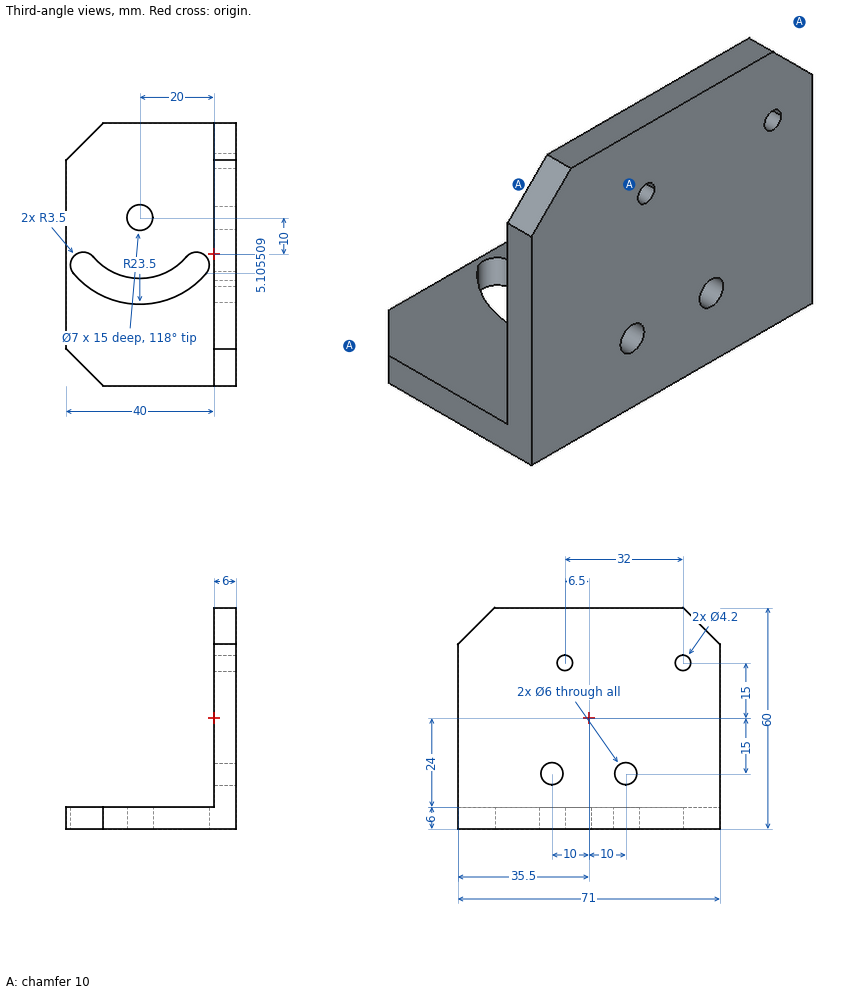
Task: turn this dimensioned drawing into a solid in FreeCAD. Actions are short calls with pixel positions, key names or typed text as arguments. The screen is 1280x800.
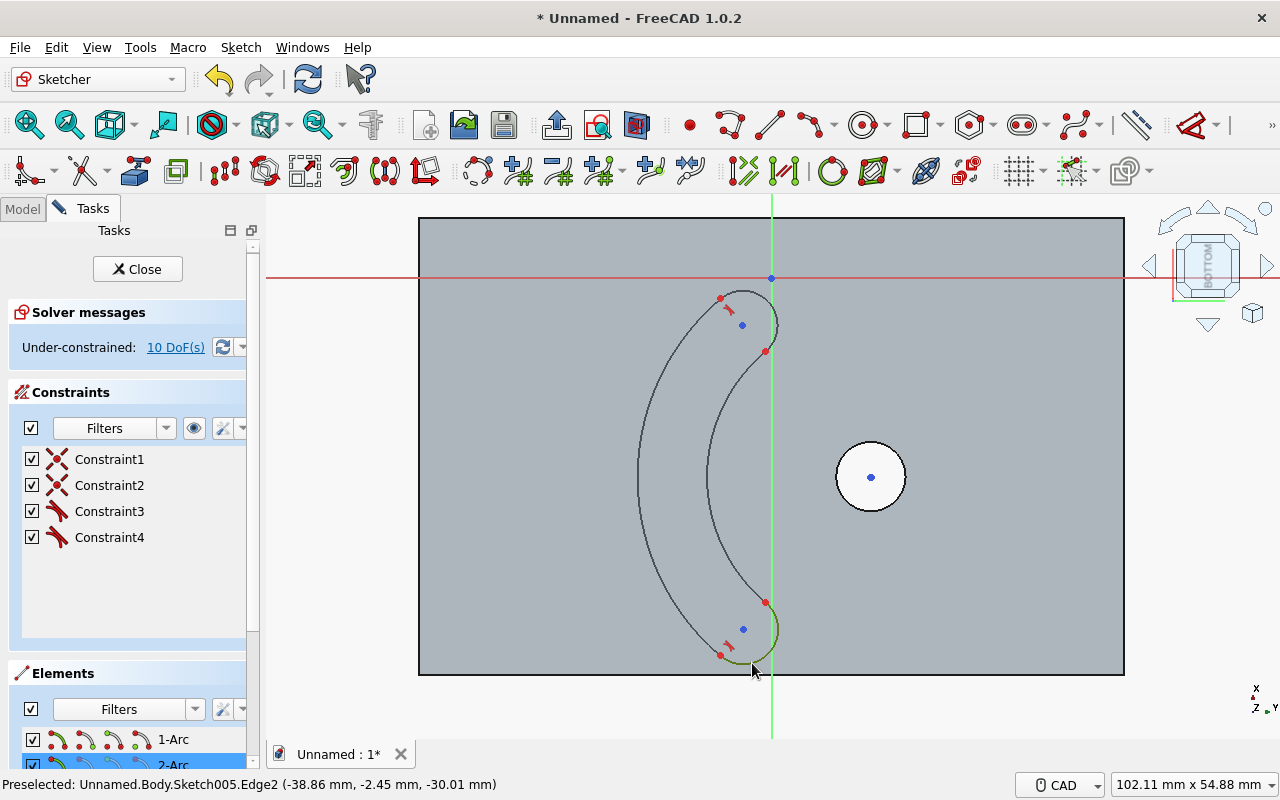
click(717, 421)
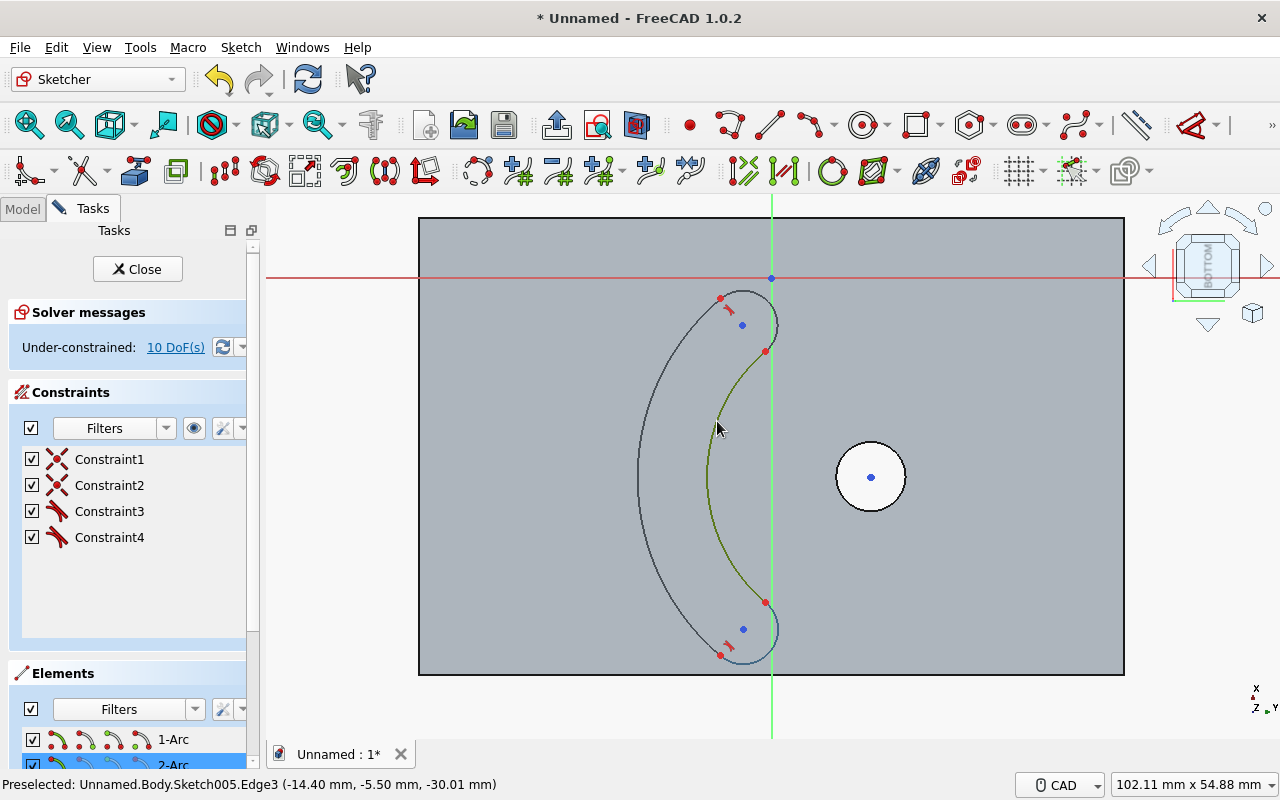
key(t)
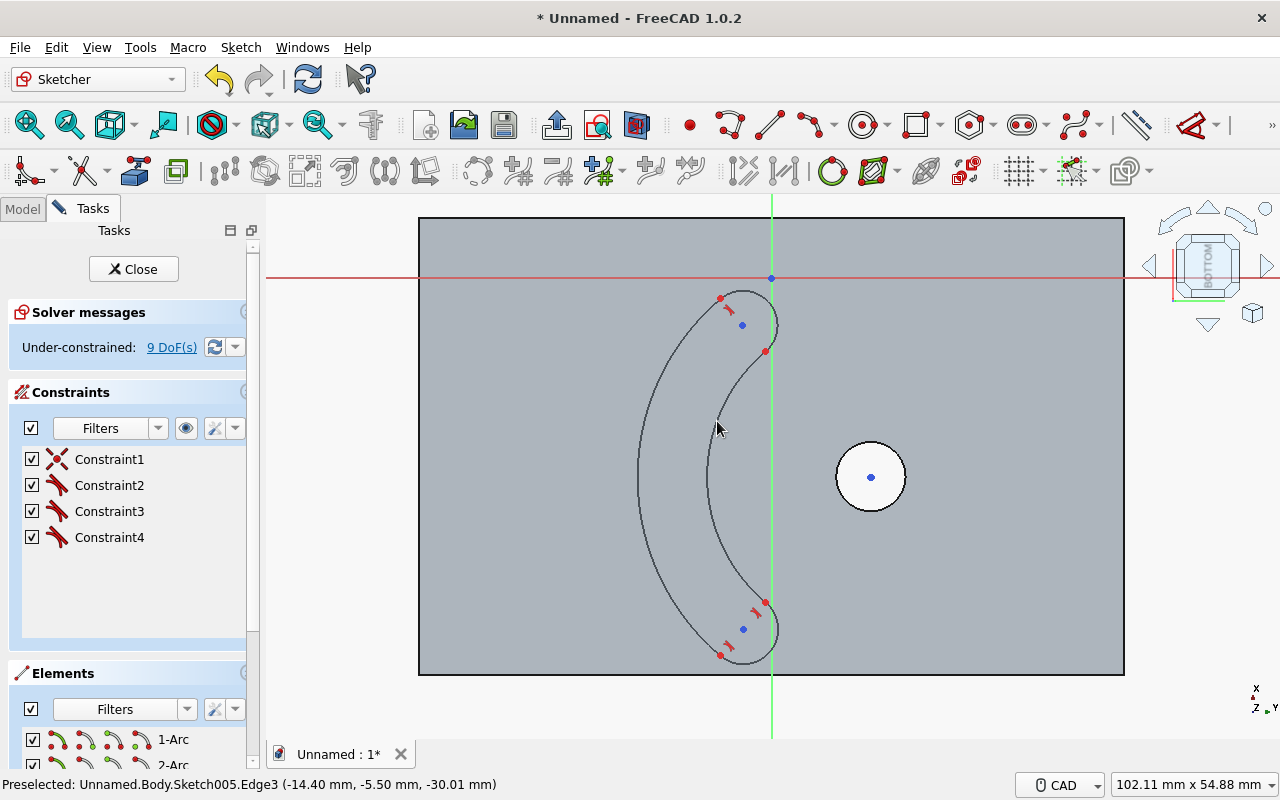
click(717, 421)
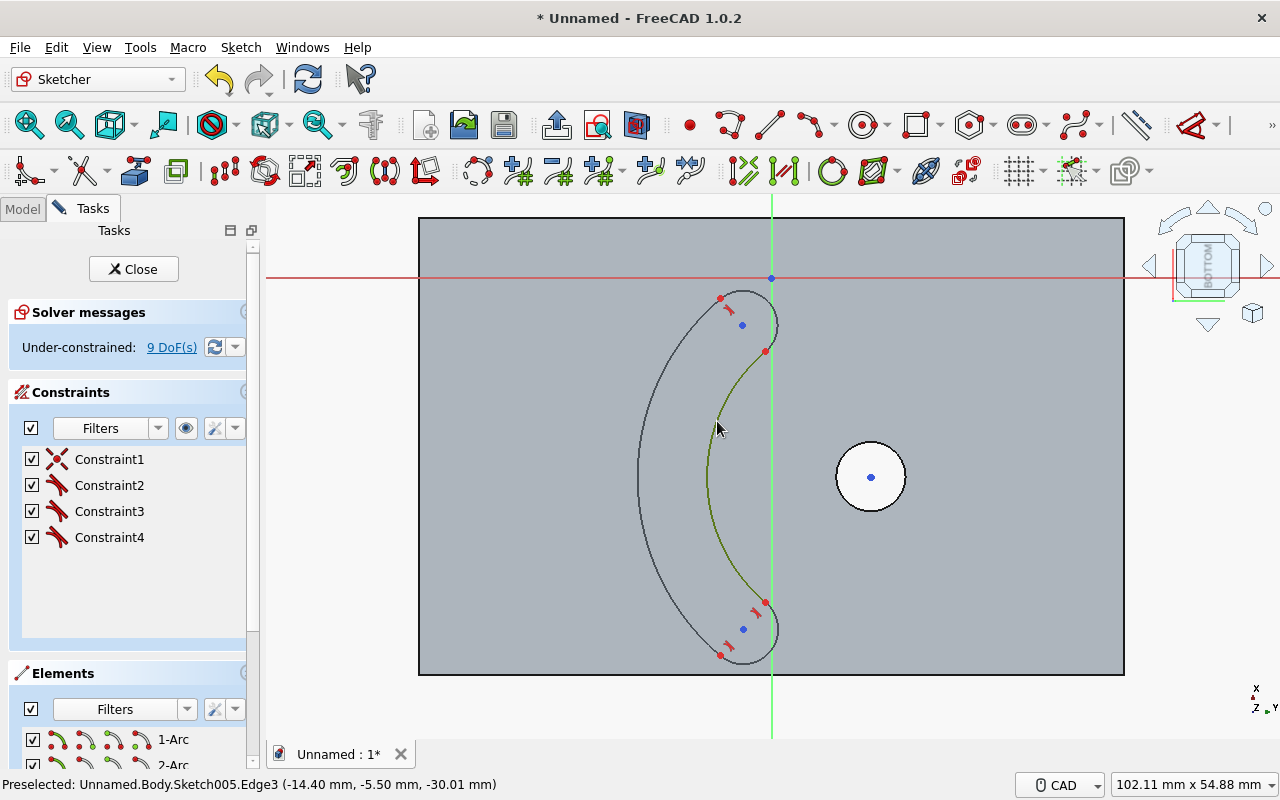
click(751, 292)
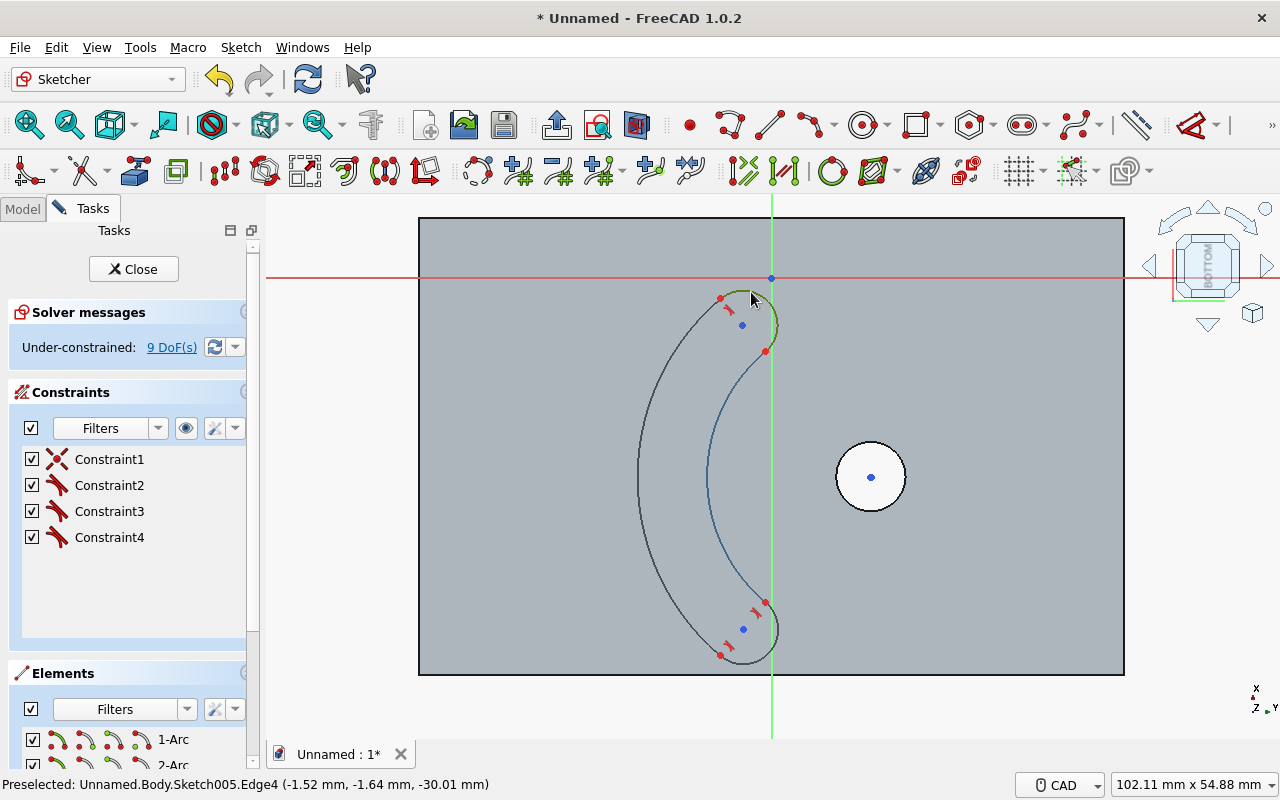
key(t)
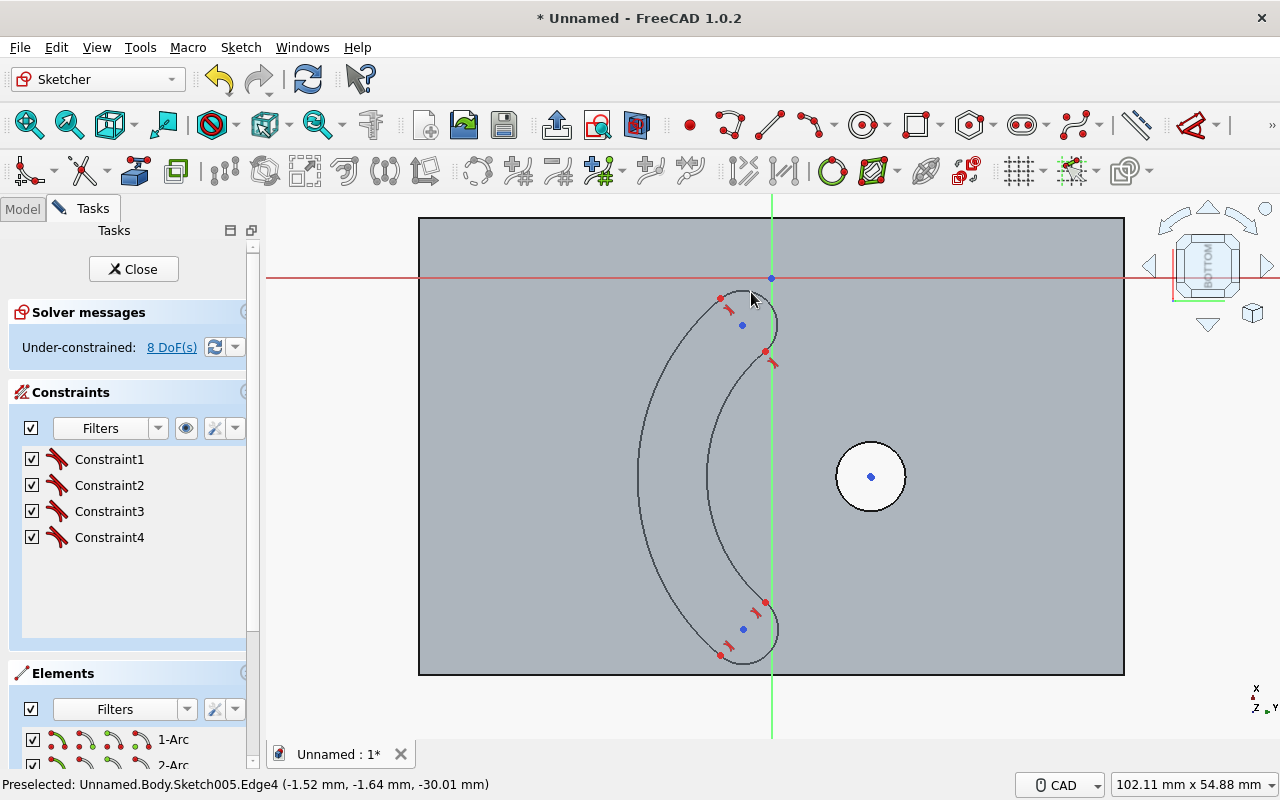
click(652, 398)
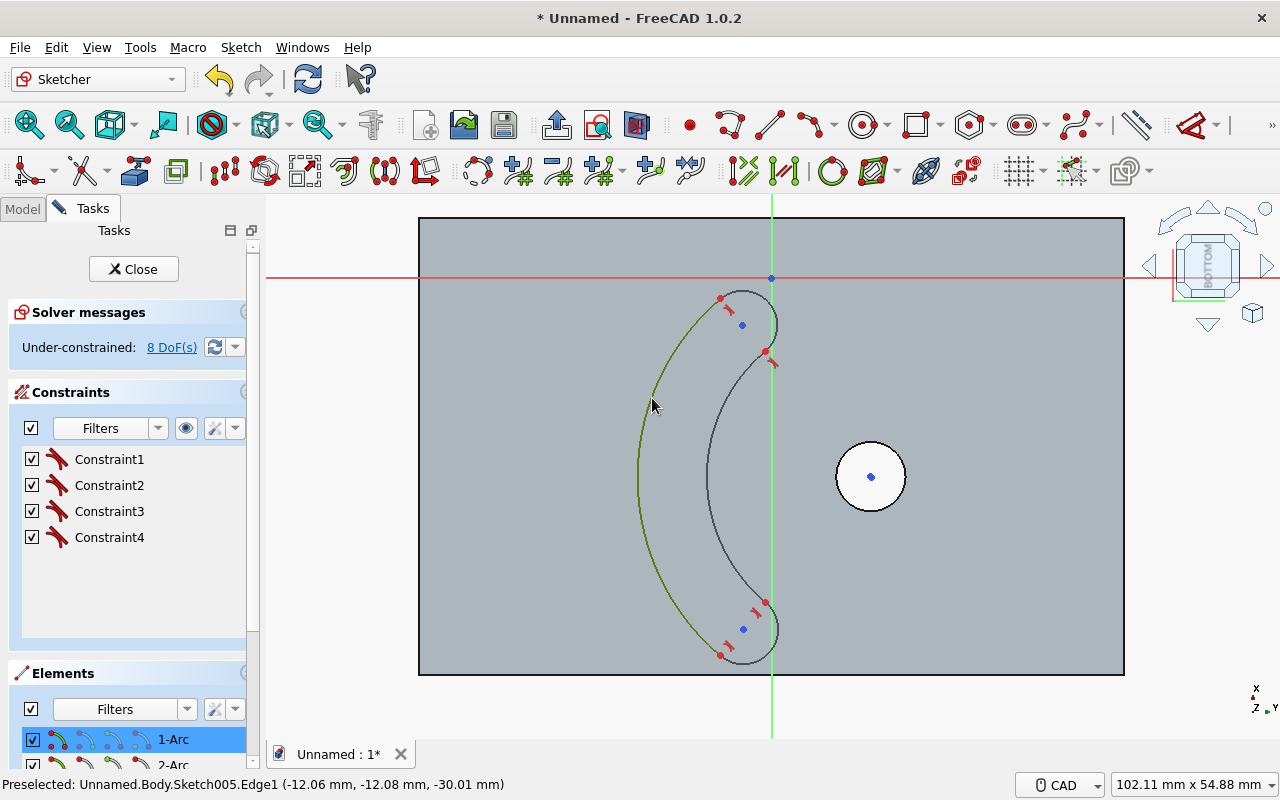
click(717, 421)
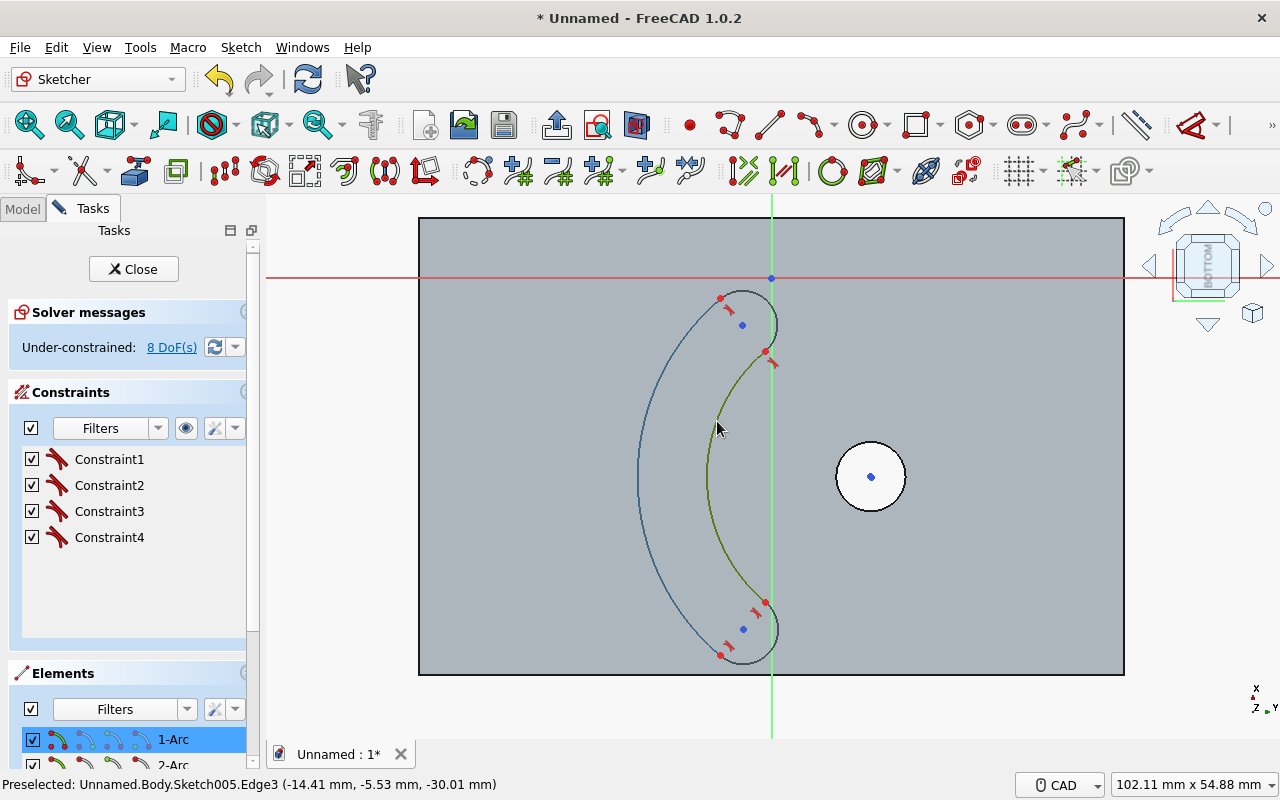
key(c)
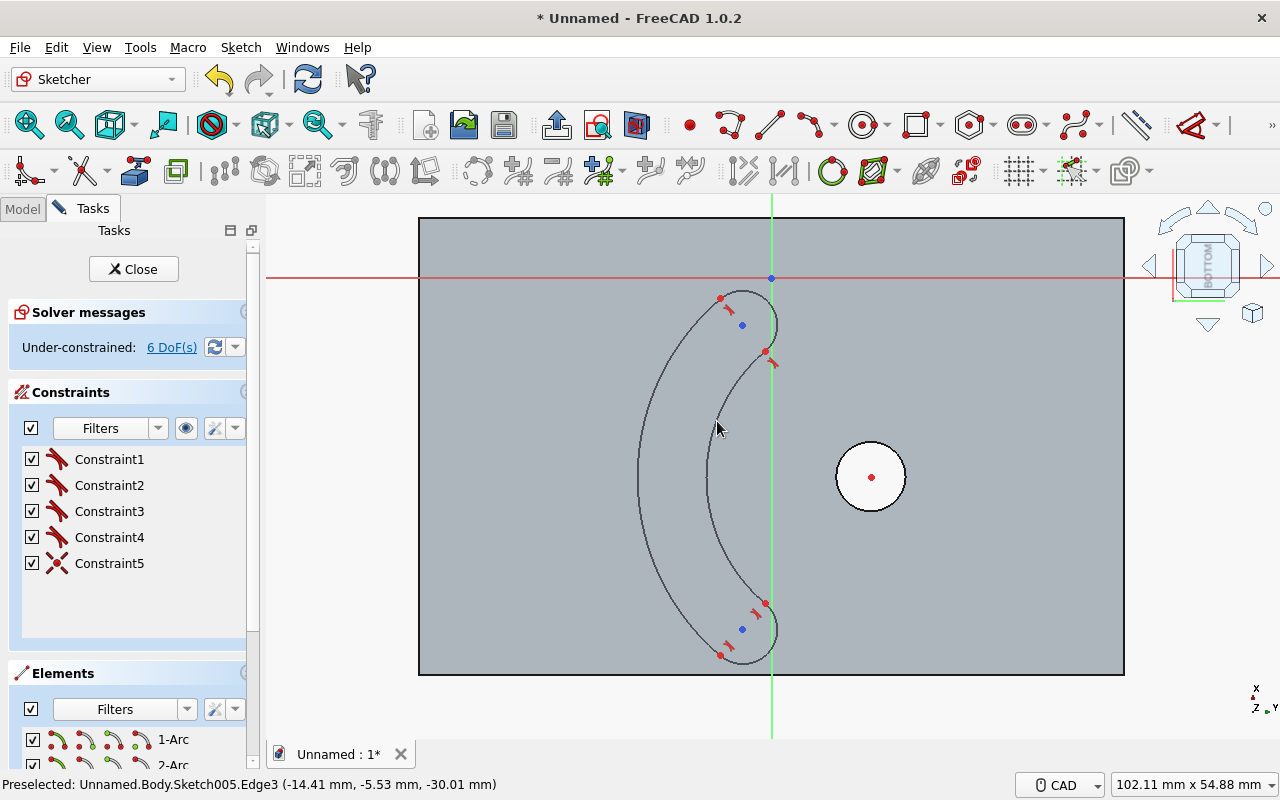
click(1192, 126)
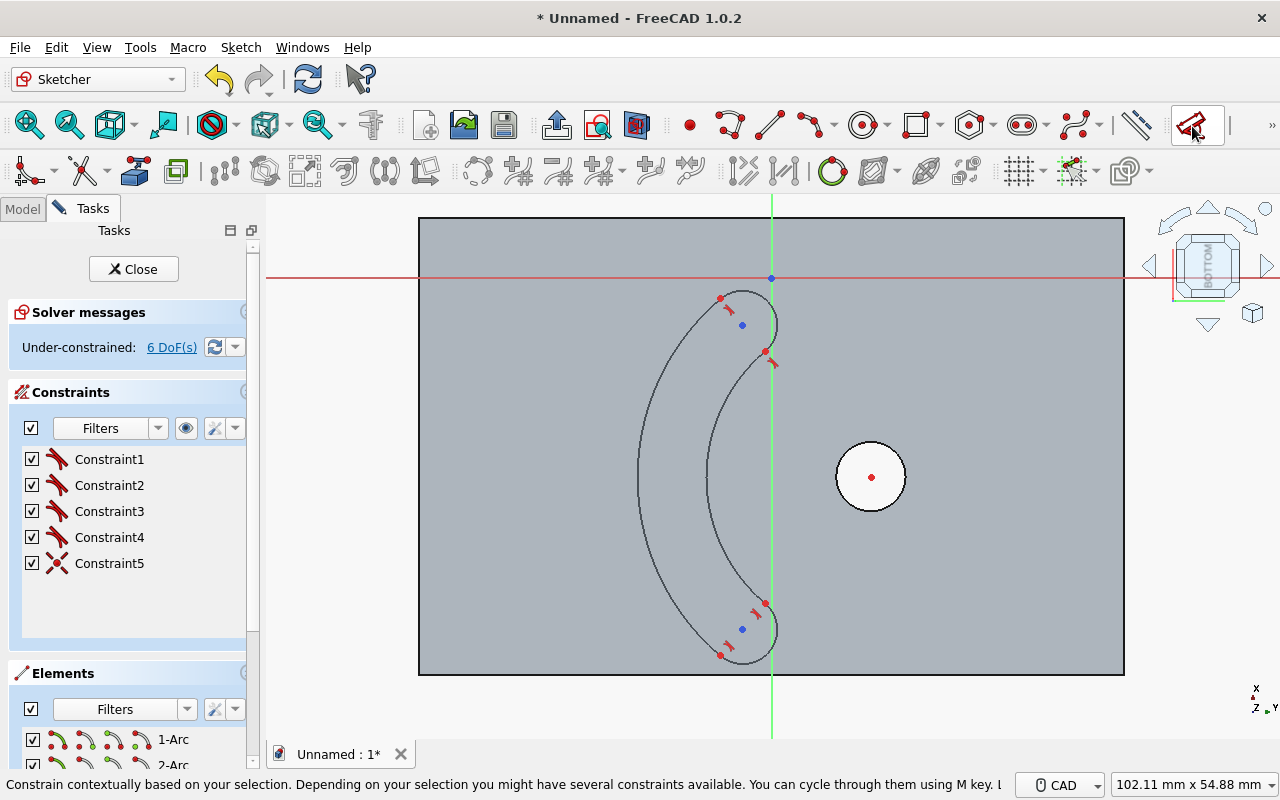
click(652, 398)
click(622, 387)